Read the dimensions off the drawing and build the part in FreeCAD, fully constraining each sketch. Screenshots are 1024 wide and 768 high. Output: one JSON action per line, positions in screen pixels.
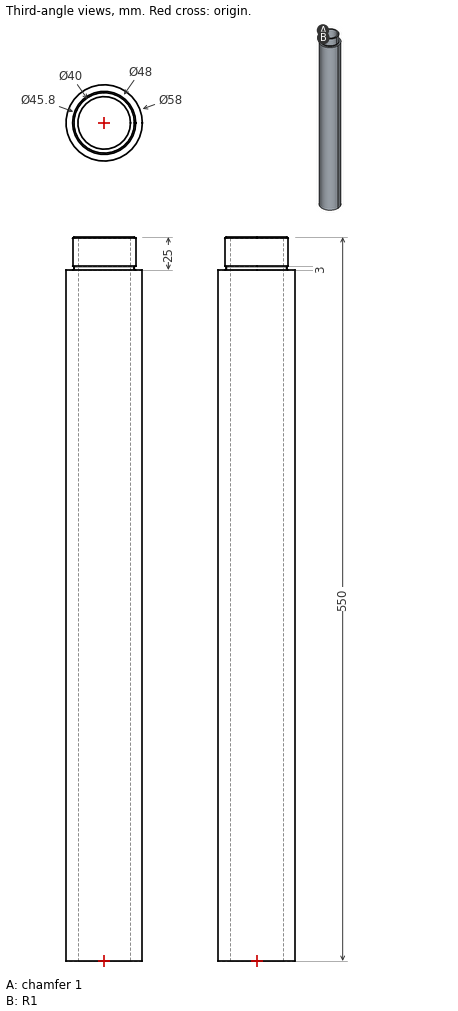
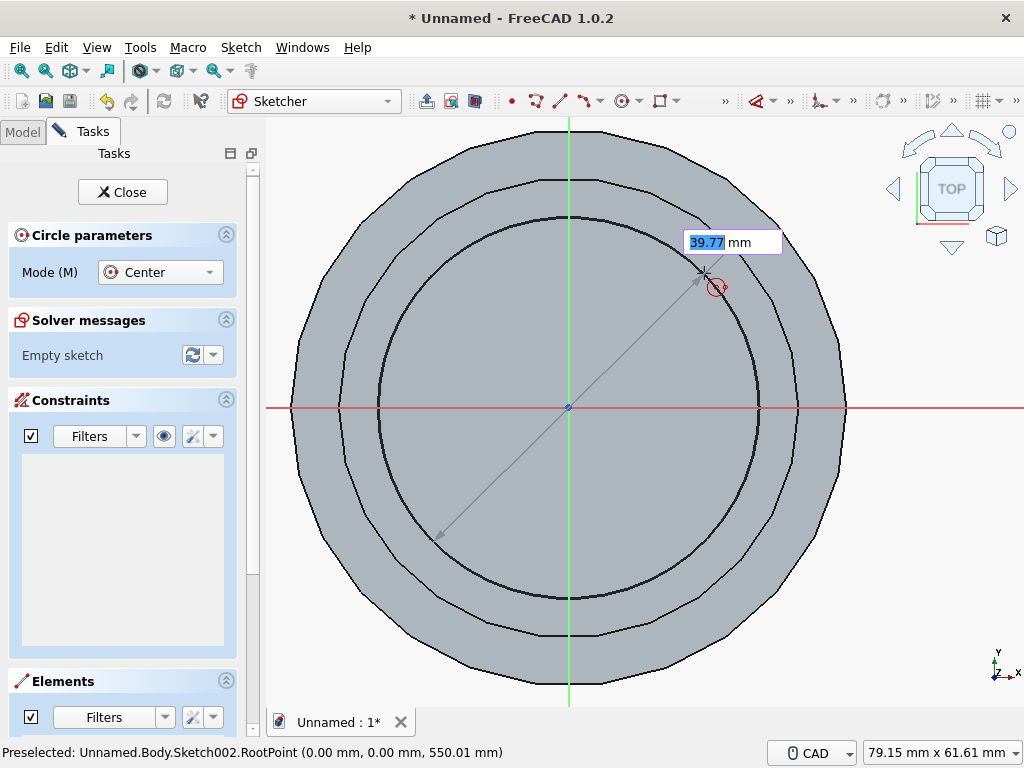
{"action": "type", "text": "40"}
{"action": "key", "text": "Return"}
{"action": "key", "text": "Escape"}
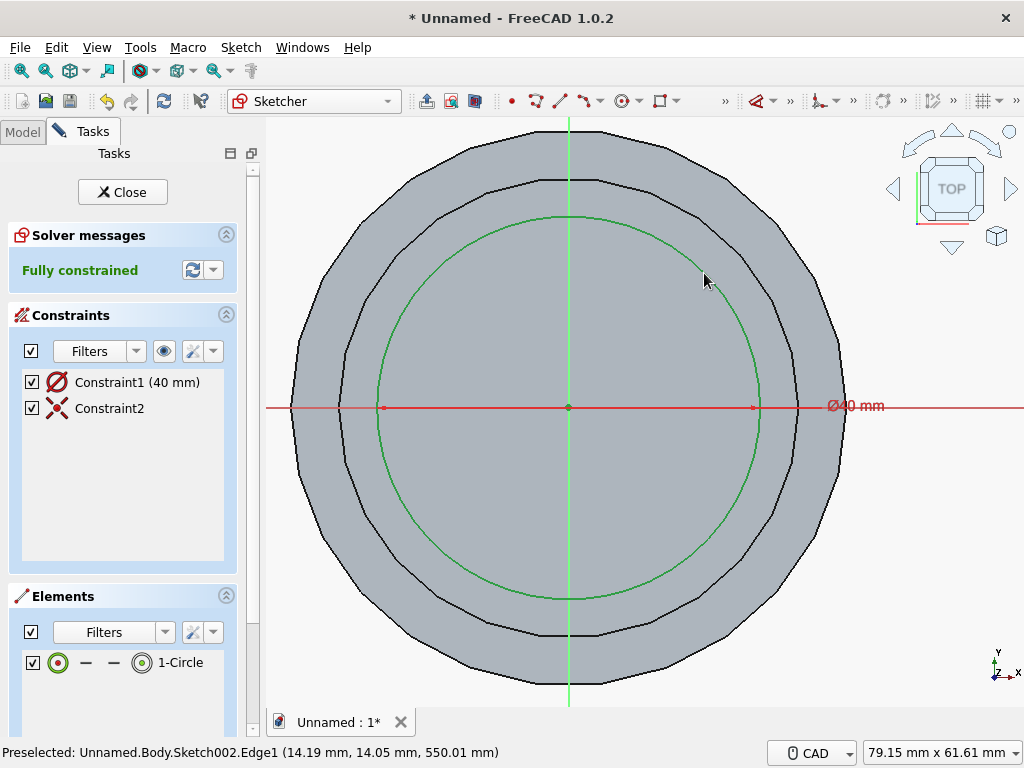
{"action": "left_click", "coordinate": [123, 192]}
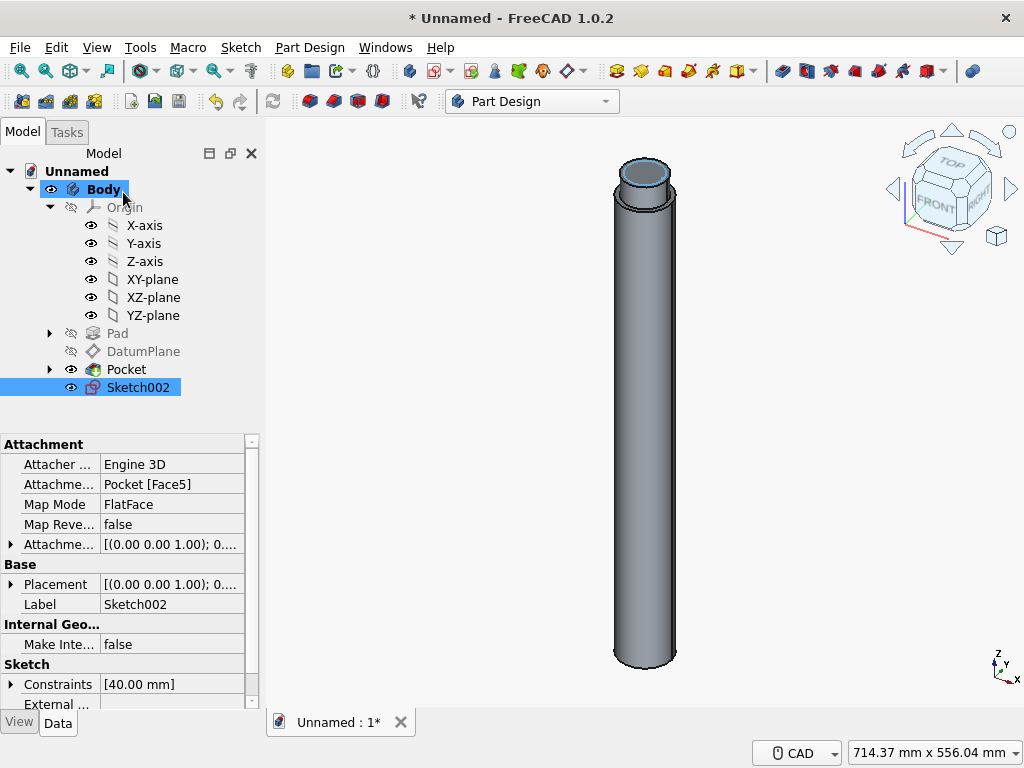
{"action": "left_click", "coordinate": [784, 72]}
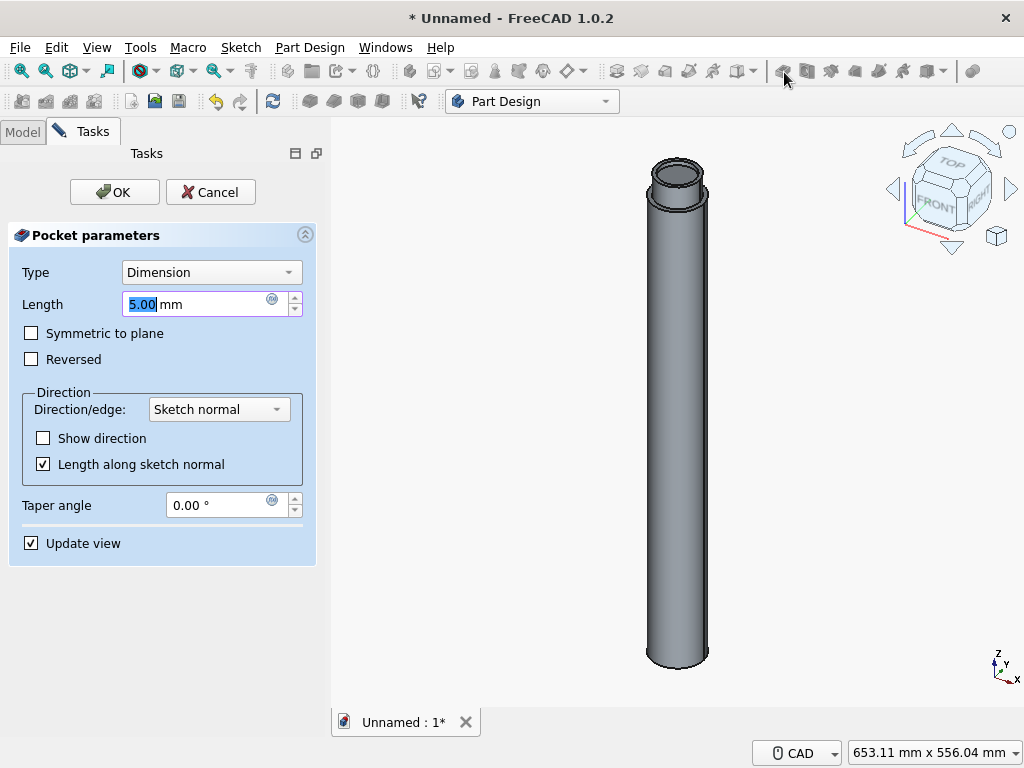
{"action": "left_click", "coordinate": [212, 272]}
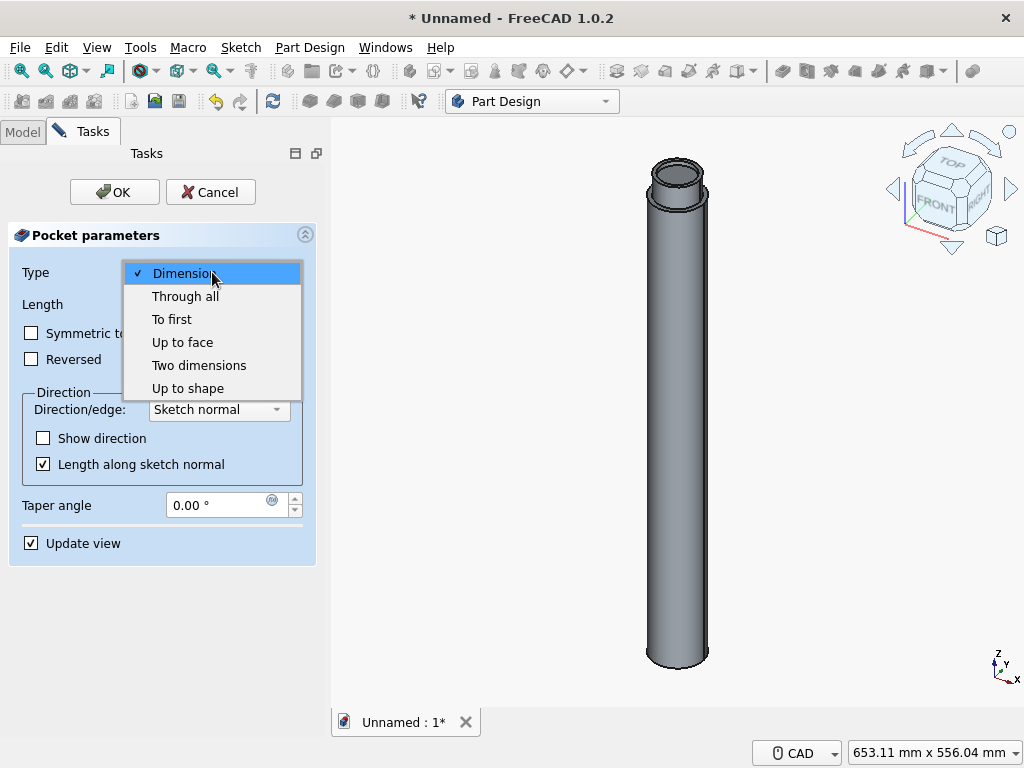
{"action": "left_click", "coordinate": [212, 296]}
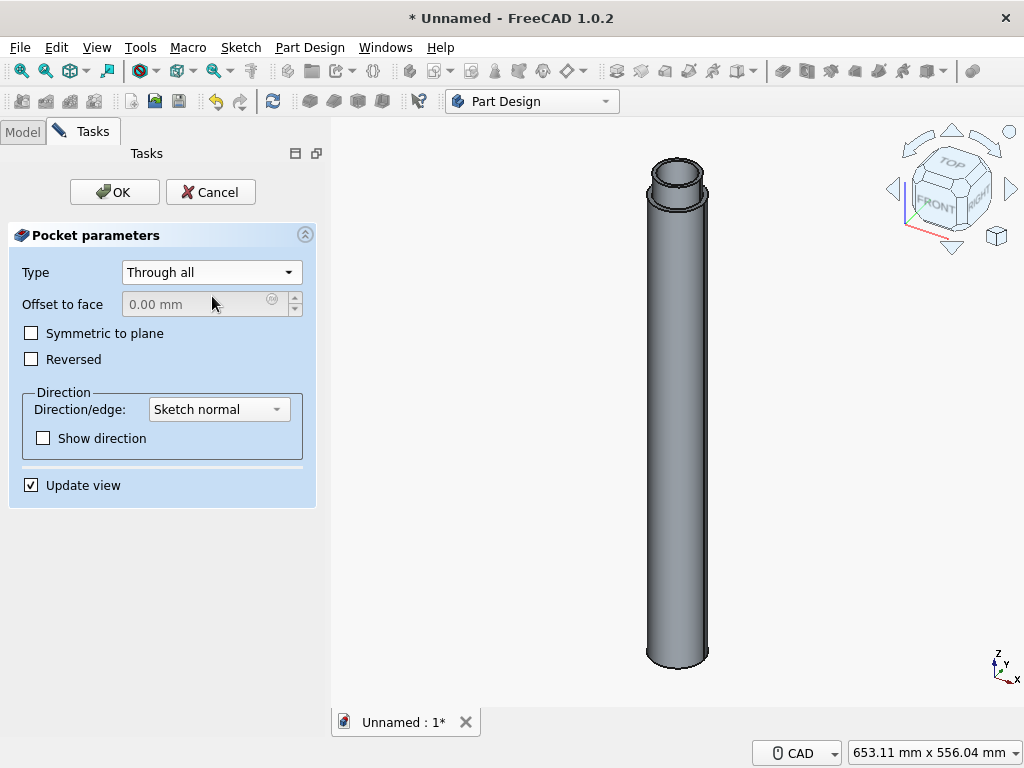
{"action": "left_click", "coordinate": [115, 192]}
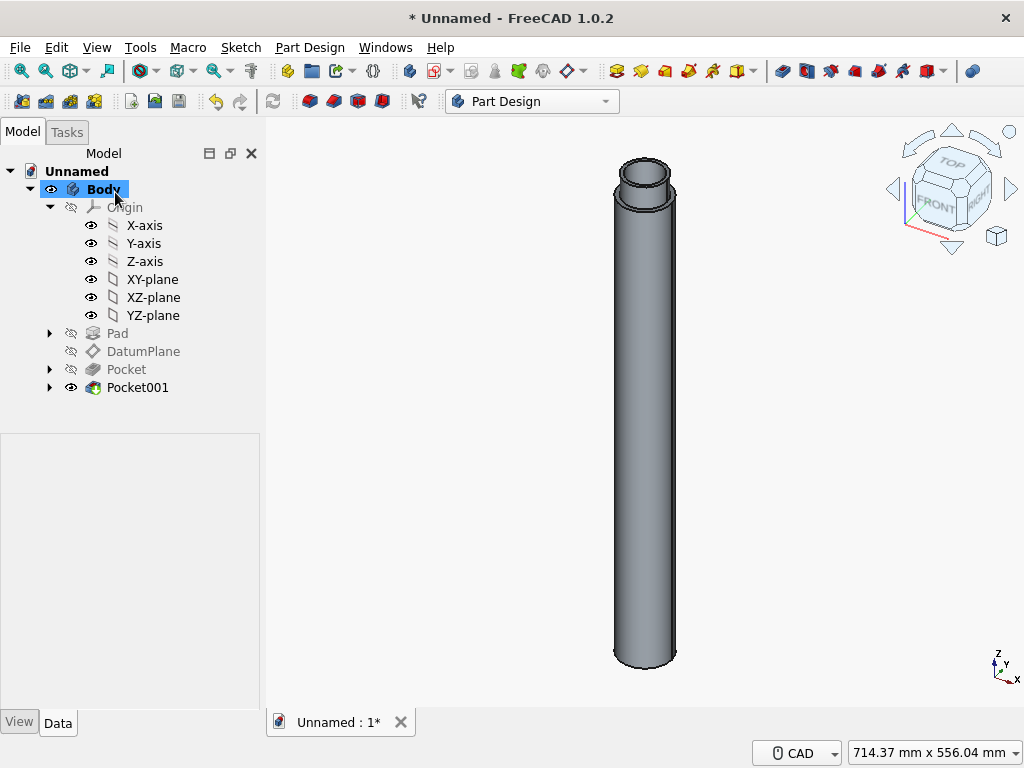
{"action": "left_click", "coordinate": [620, 174]}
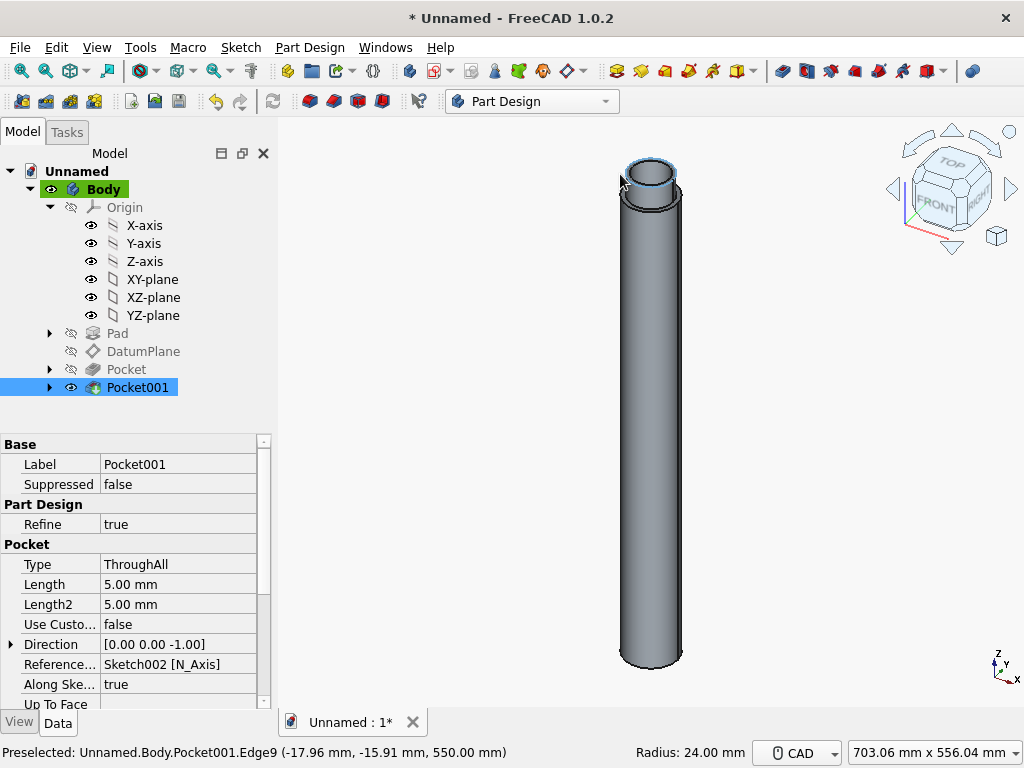
{"action": "left_click", "coordinate": [334, 102]}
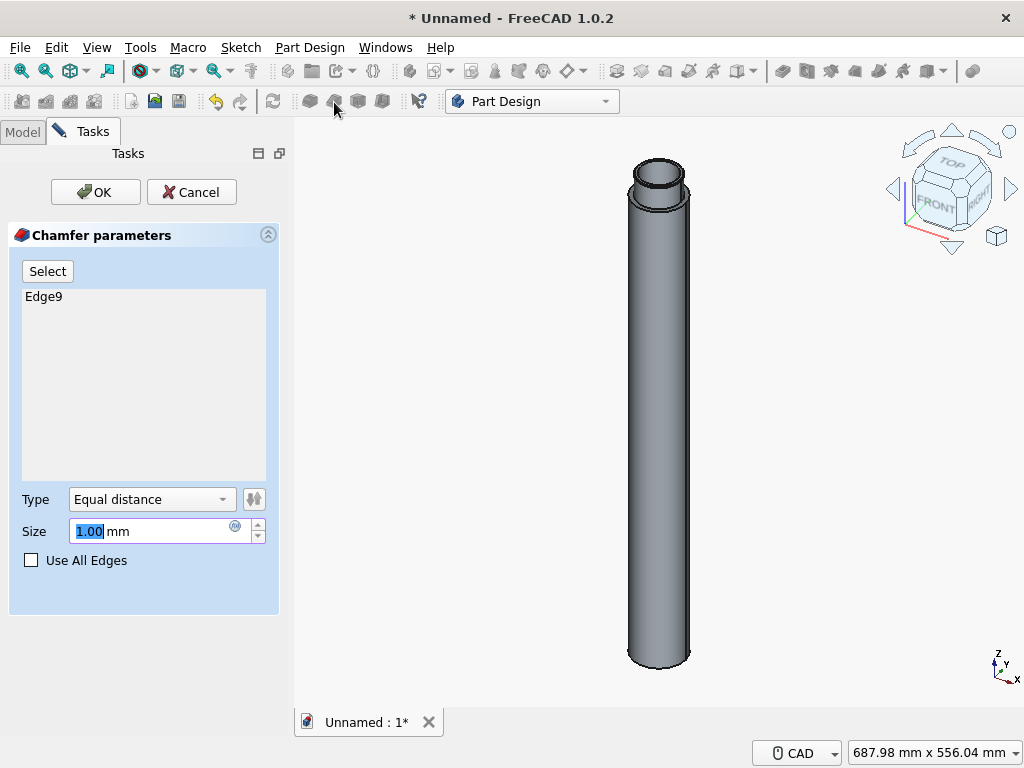
{"action": "type", "text": "1"}
{"action": "key", "text": "Tab"}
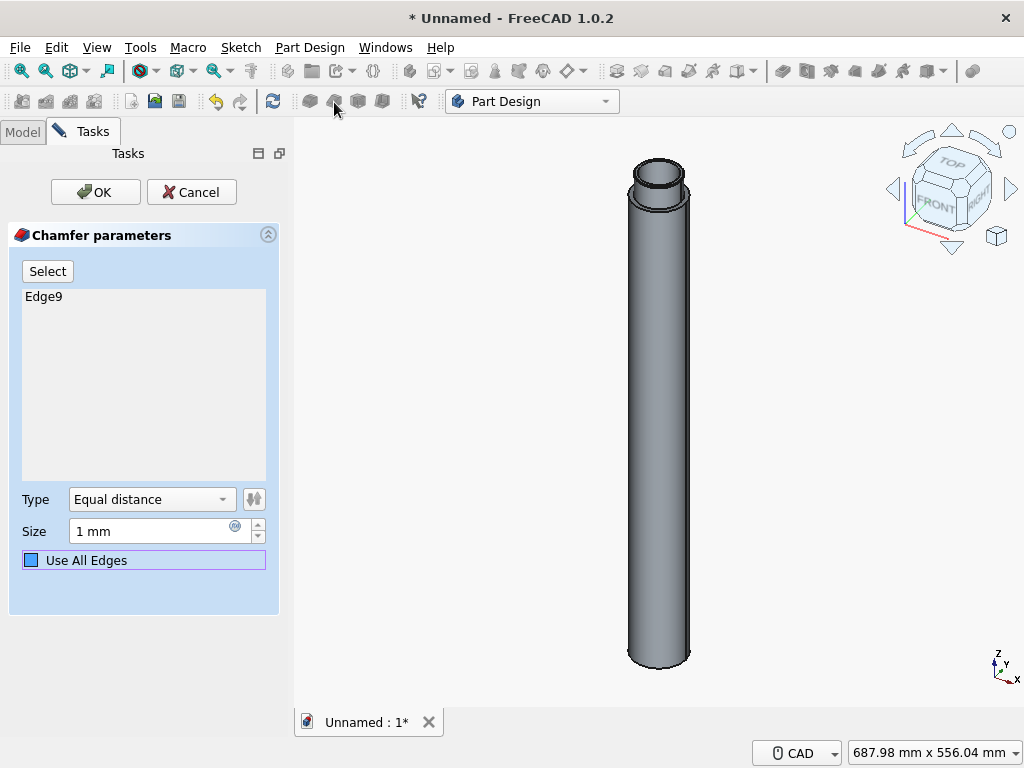
{"action": "left_click", "coordinate": [96, 192]}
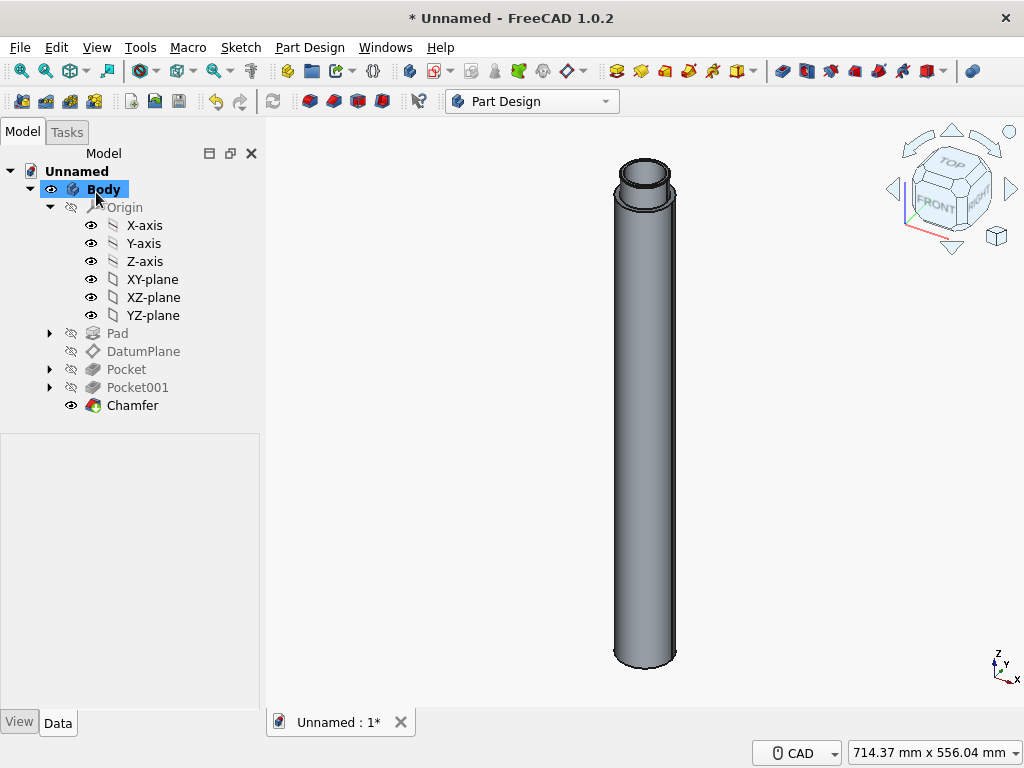
{"action": "scroll", "coordinate": [624, 204], "scroll_direction": "up", "scroll_amount": 9}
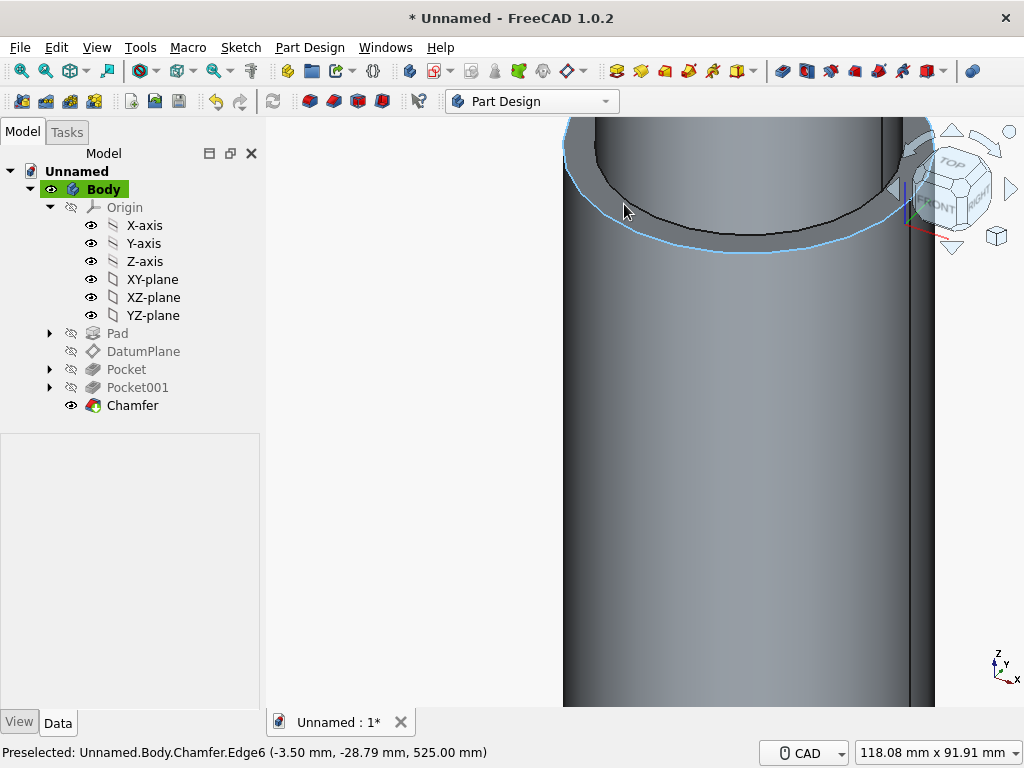
{"action": "left_click", "coordinate": [623, 210]}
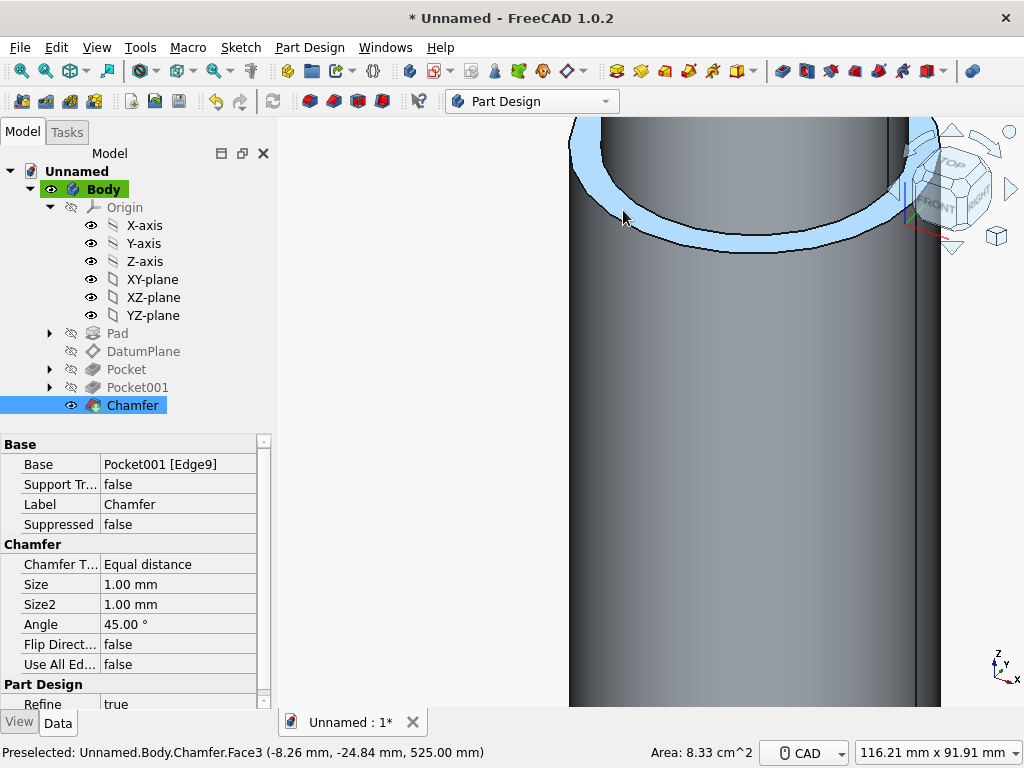
{"action": "left_click", "coordinate": [434, 72]}